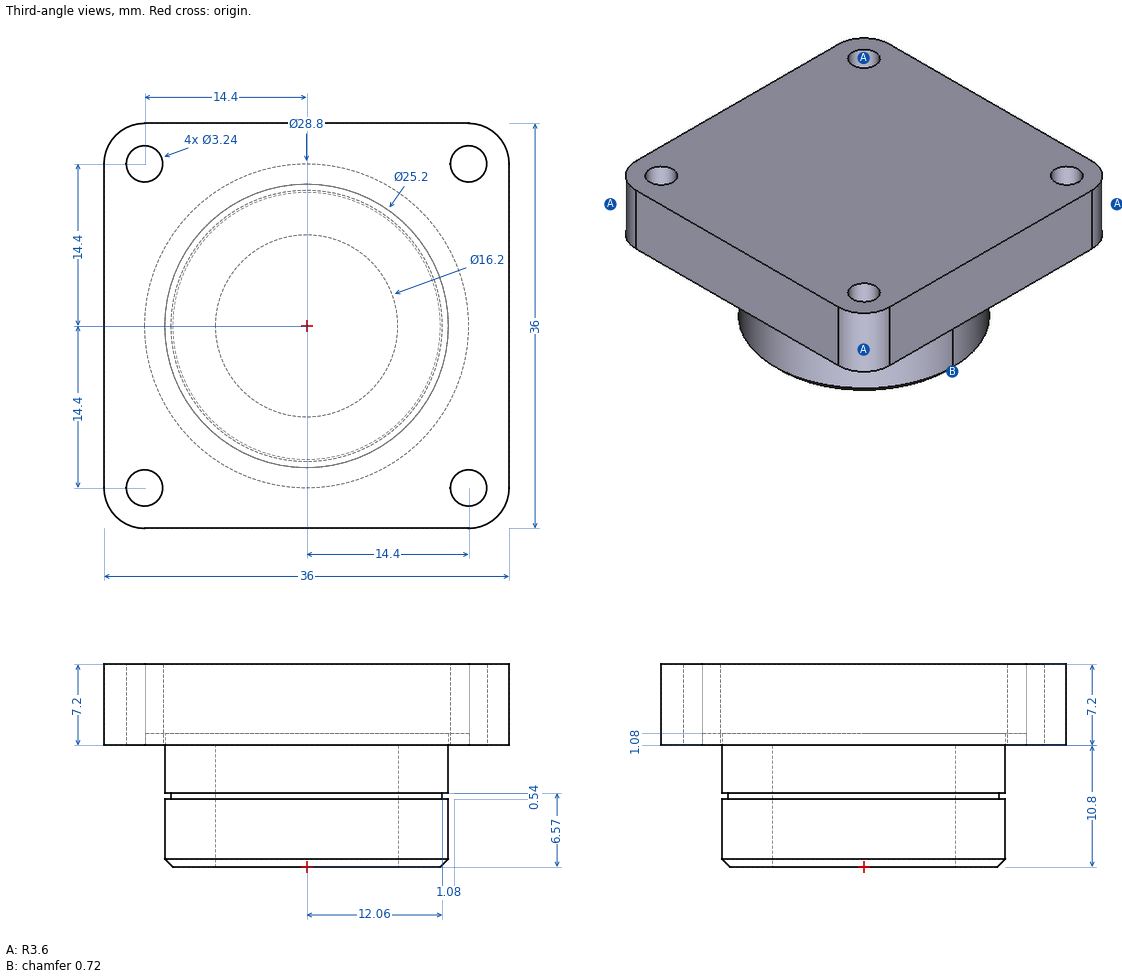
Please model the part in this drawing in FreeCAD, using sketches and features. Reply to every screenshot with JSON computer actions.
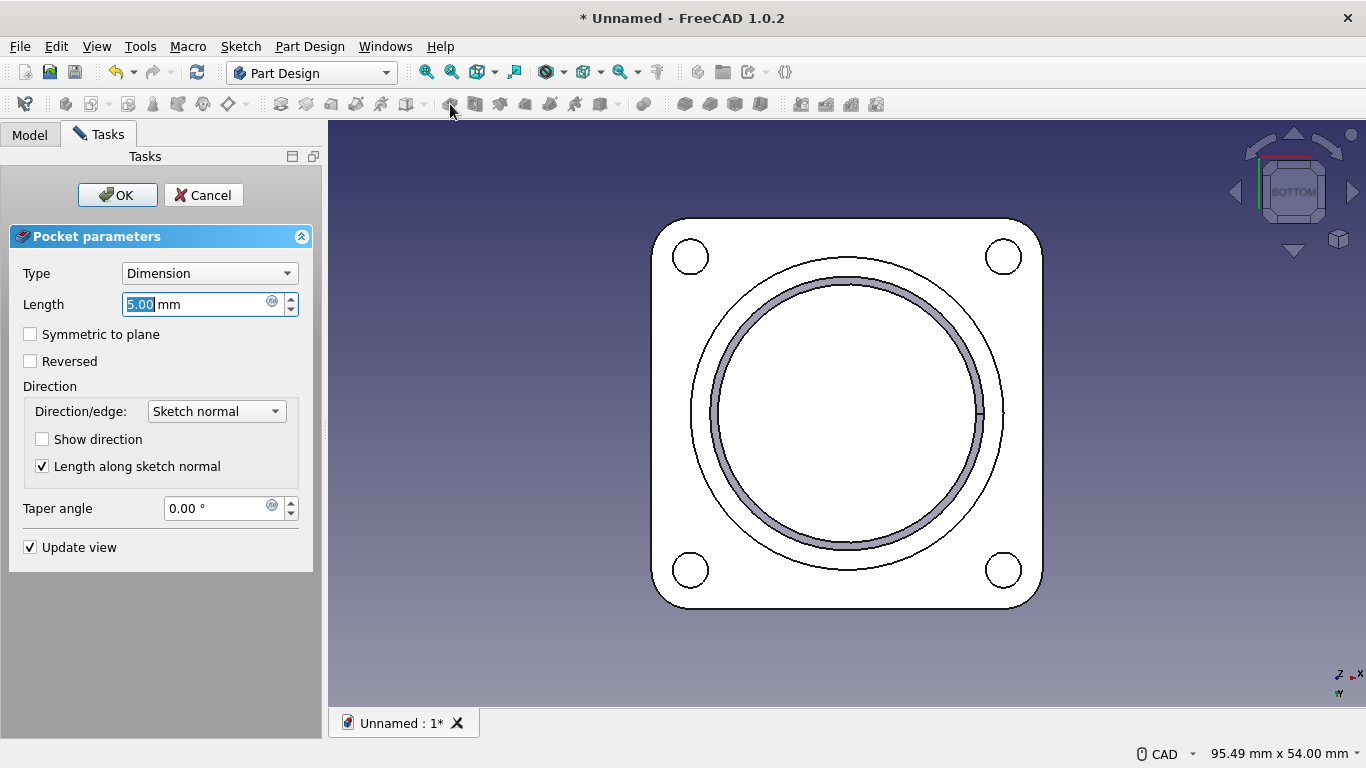
{"action": "type", "text": "7.2"}
{"action": "key", "text": "Tab"}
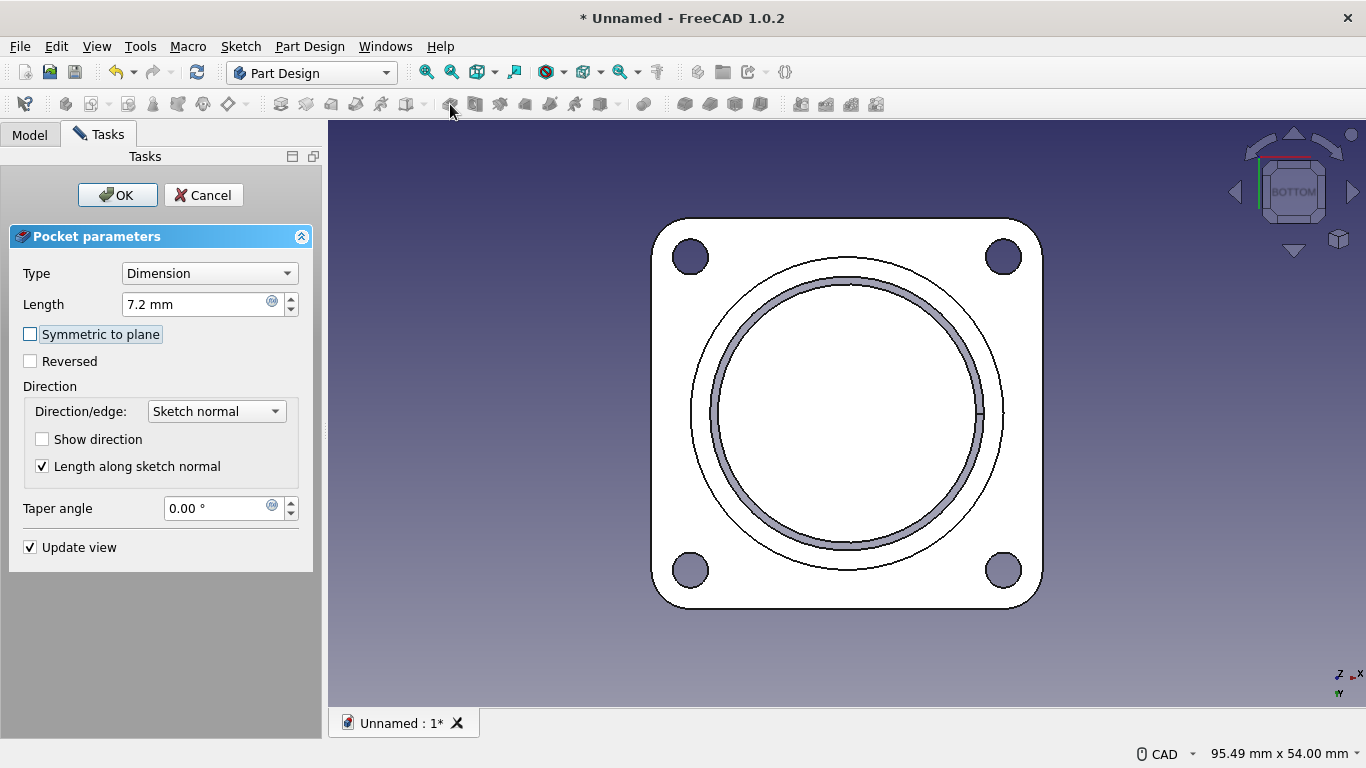
{"action": "left_click", "coordinate": [118, 195]}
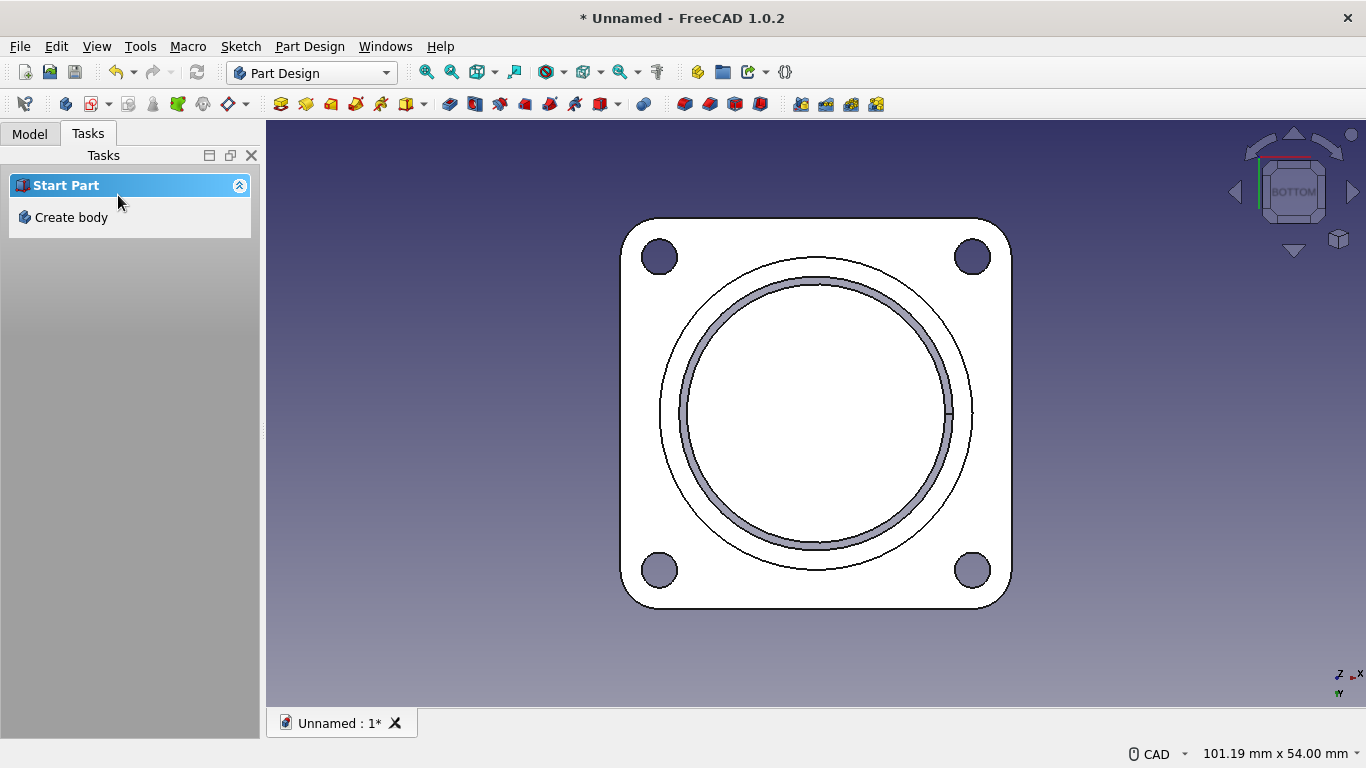
{"action": "left_click", "coordinate": [90, 104]}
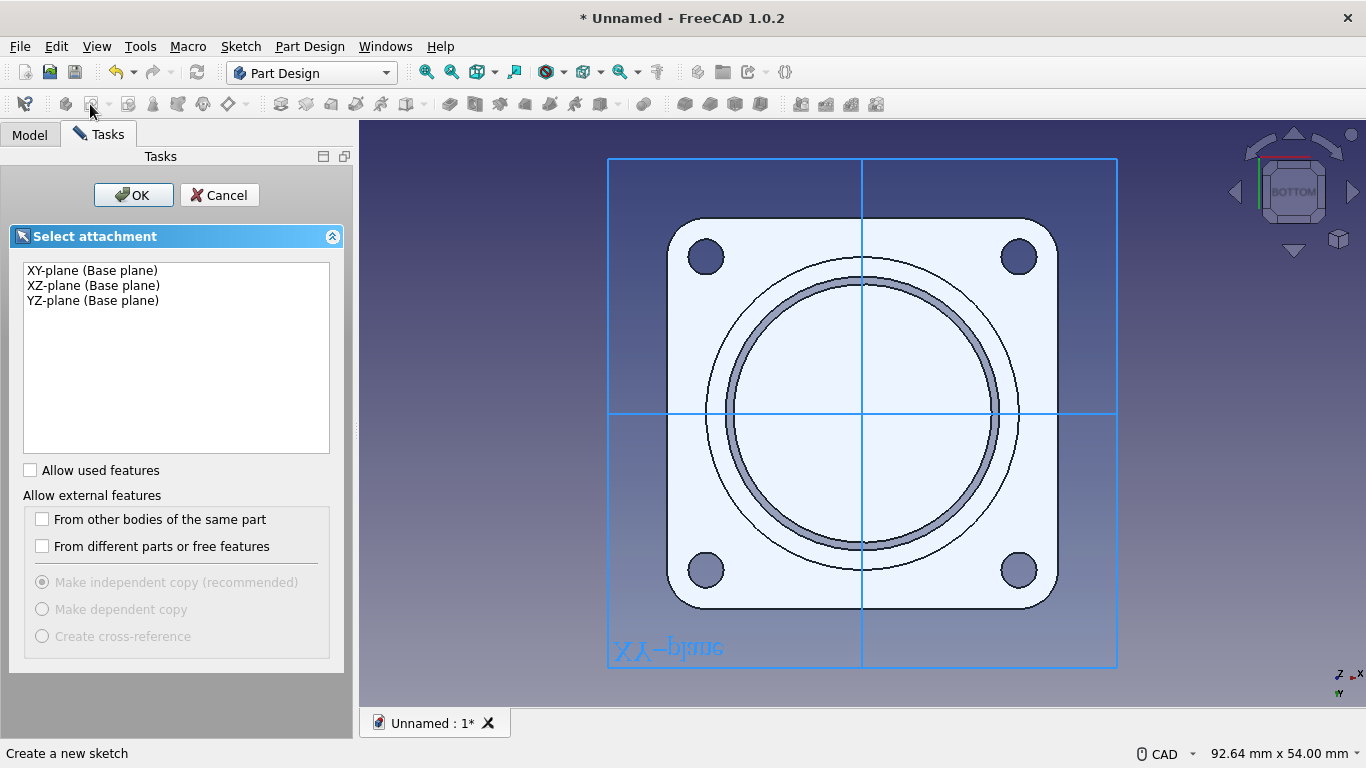
{"action": "left_click", "coordinate": [84, 270]}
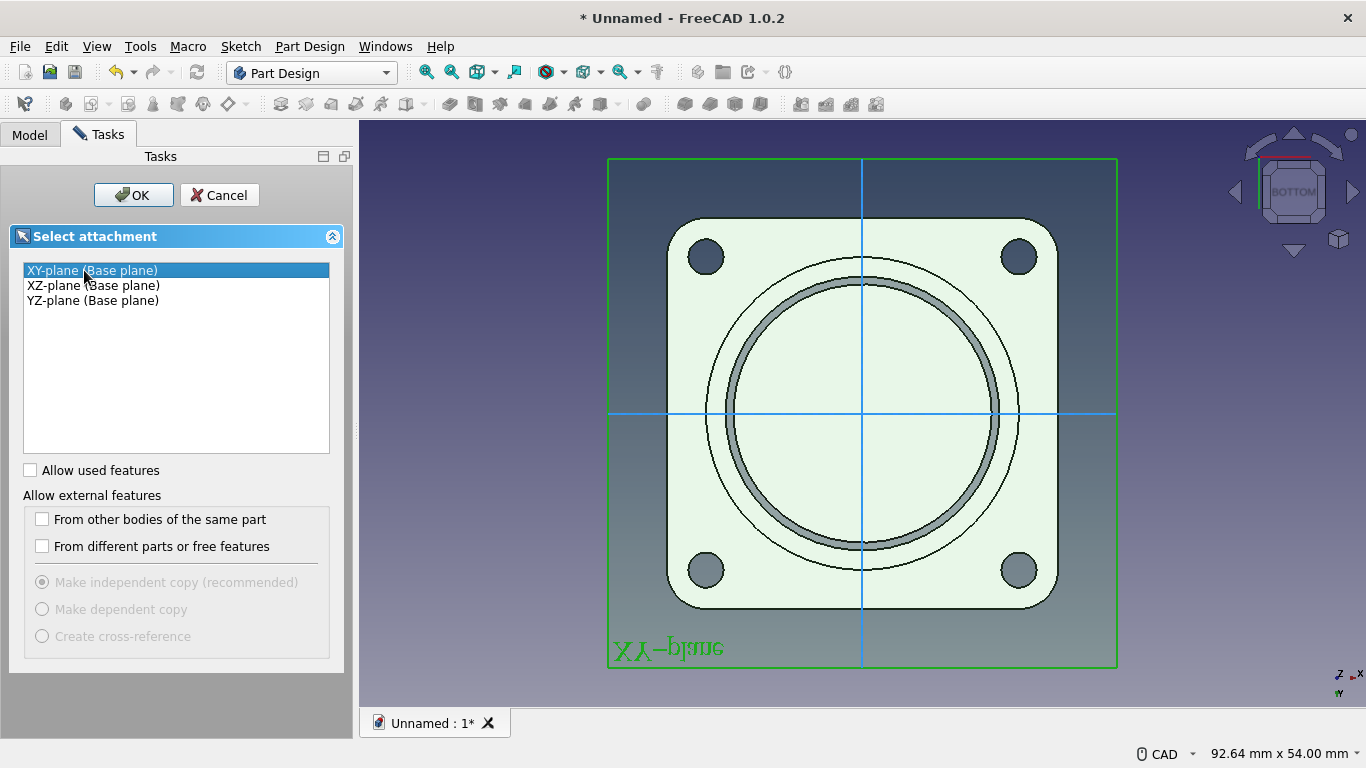
{"action": "left_click", "coordinate": [134, 195]}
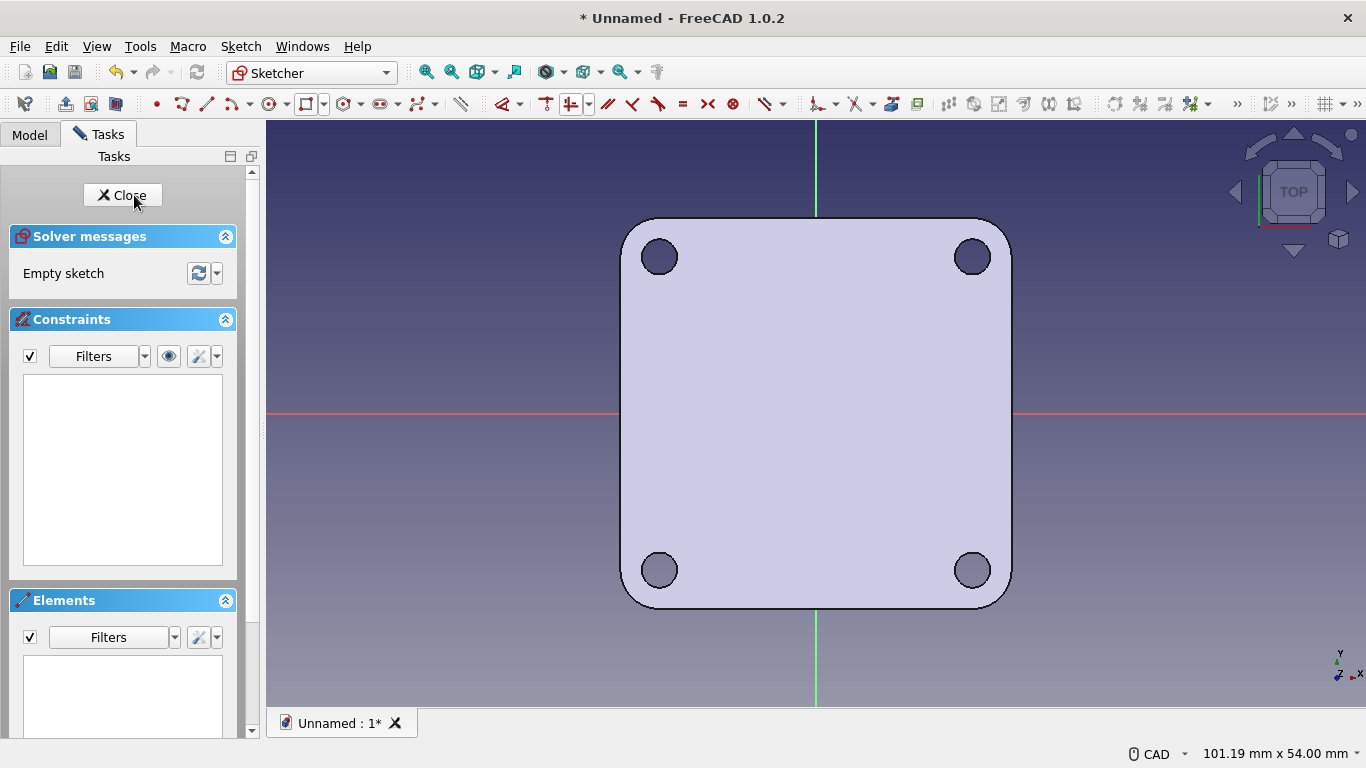
{"action": "left_click", "coordinate": [116, 104]}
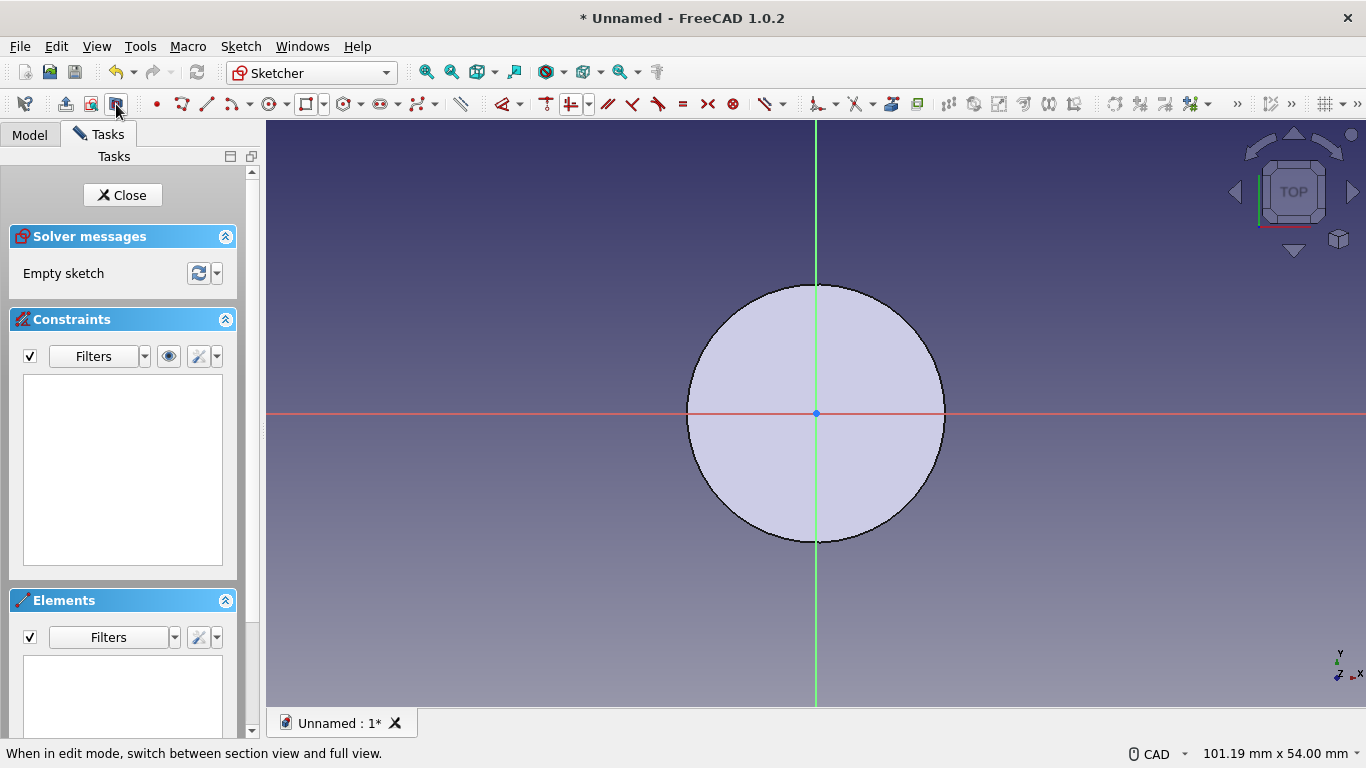
{"action": "scroll", "coordinate": [872, 413], "scroll_direction": "up", "scroll_amount": 4}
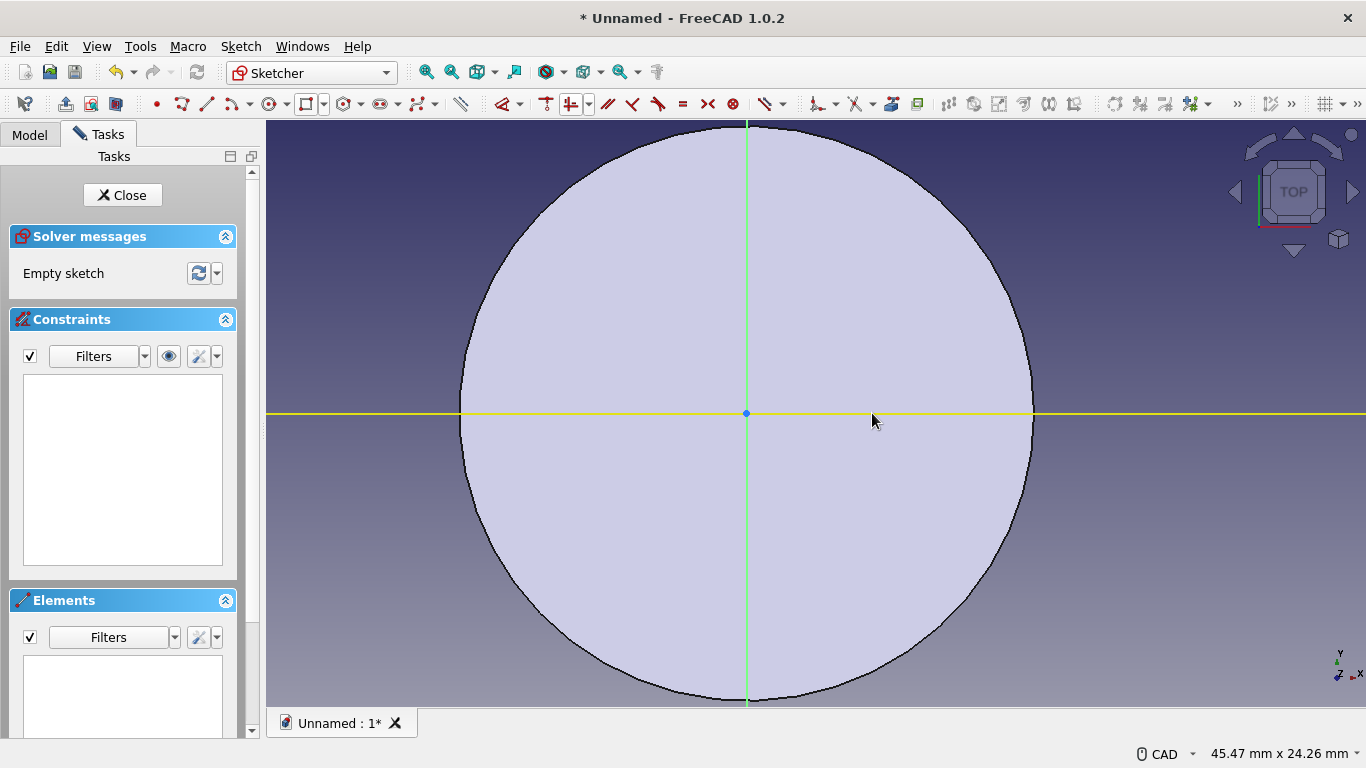
{"action": "left_click", "coordinate": [268, 104]}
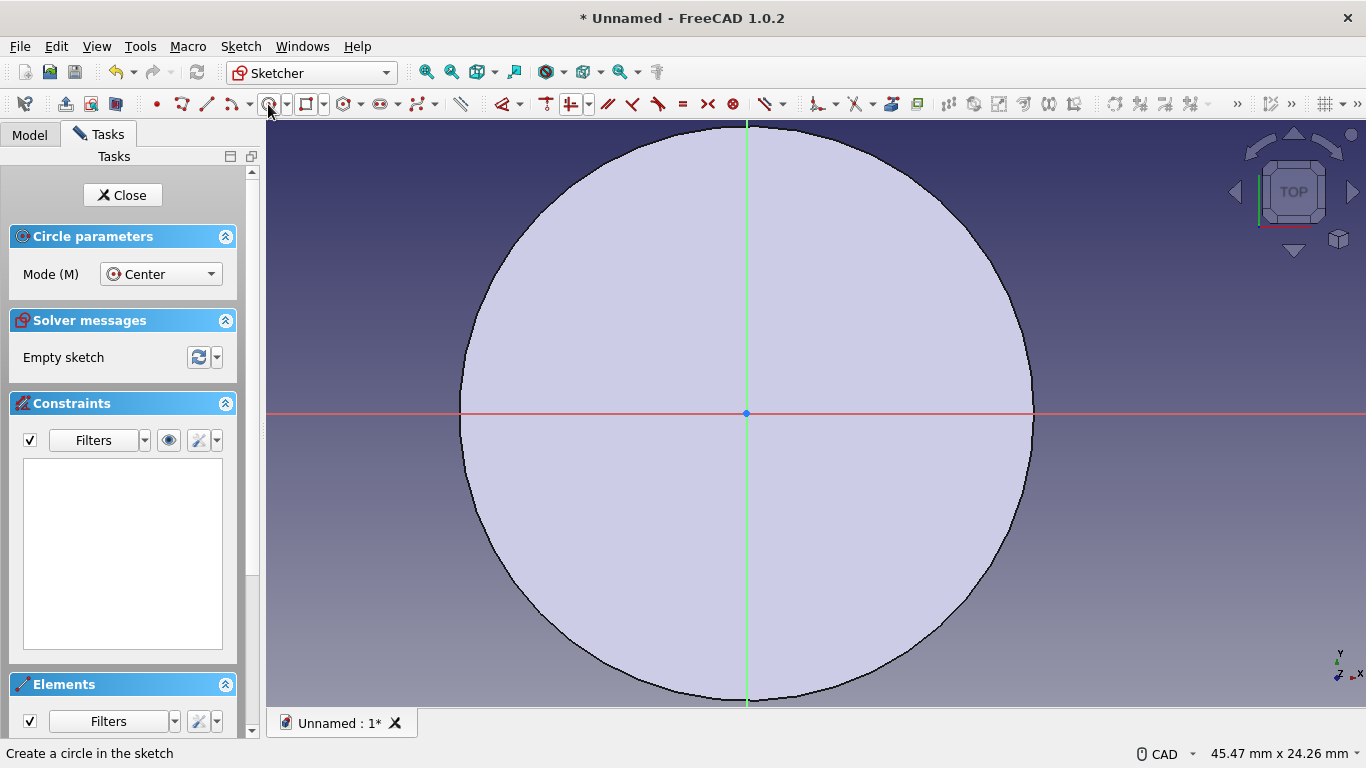
{"action": "left_click", "coordinate": [747, 413]}
{"action": "mouse_move", "coordinate": [885, 275]}